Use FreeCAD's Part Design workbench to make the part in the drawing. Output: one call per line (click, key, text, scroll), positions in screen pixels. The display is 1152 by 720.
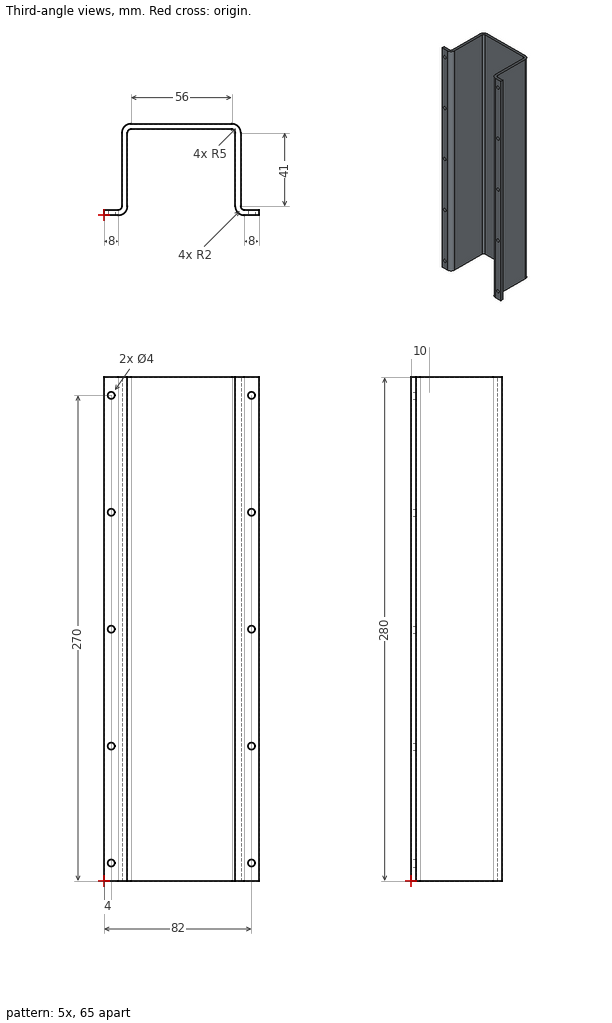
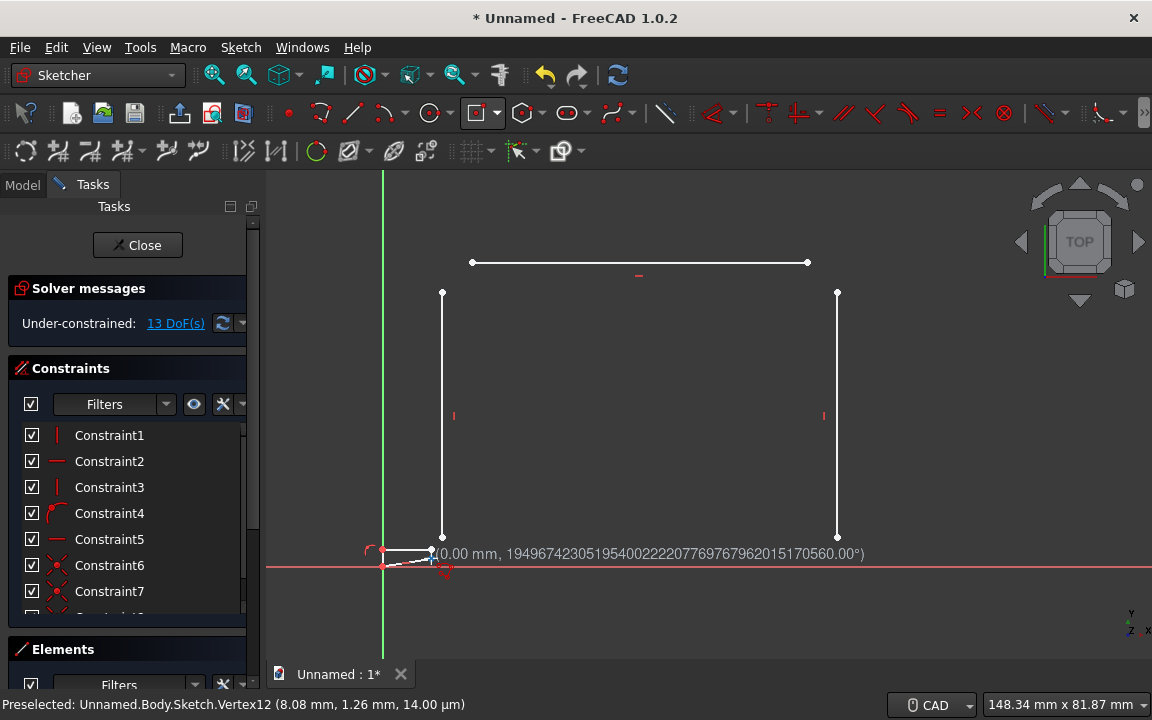
key(g)
key(l)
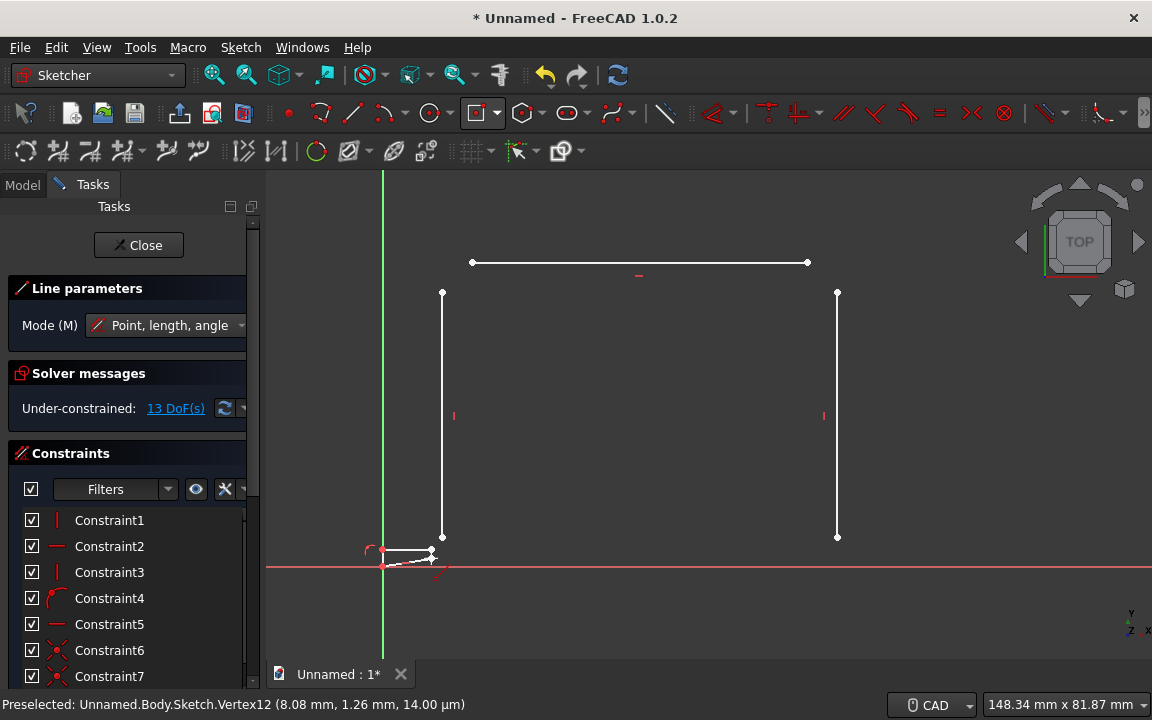
click(460, 537)
click(460, 292)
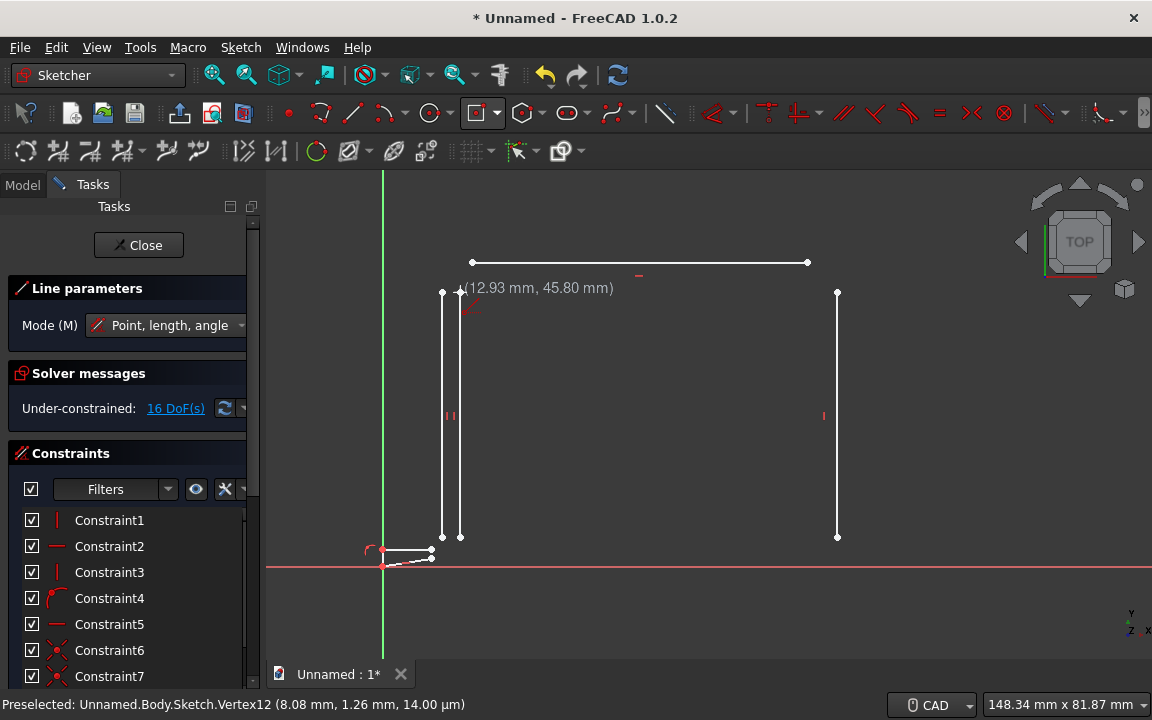
click(472, 280)
click(807, 280)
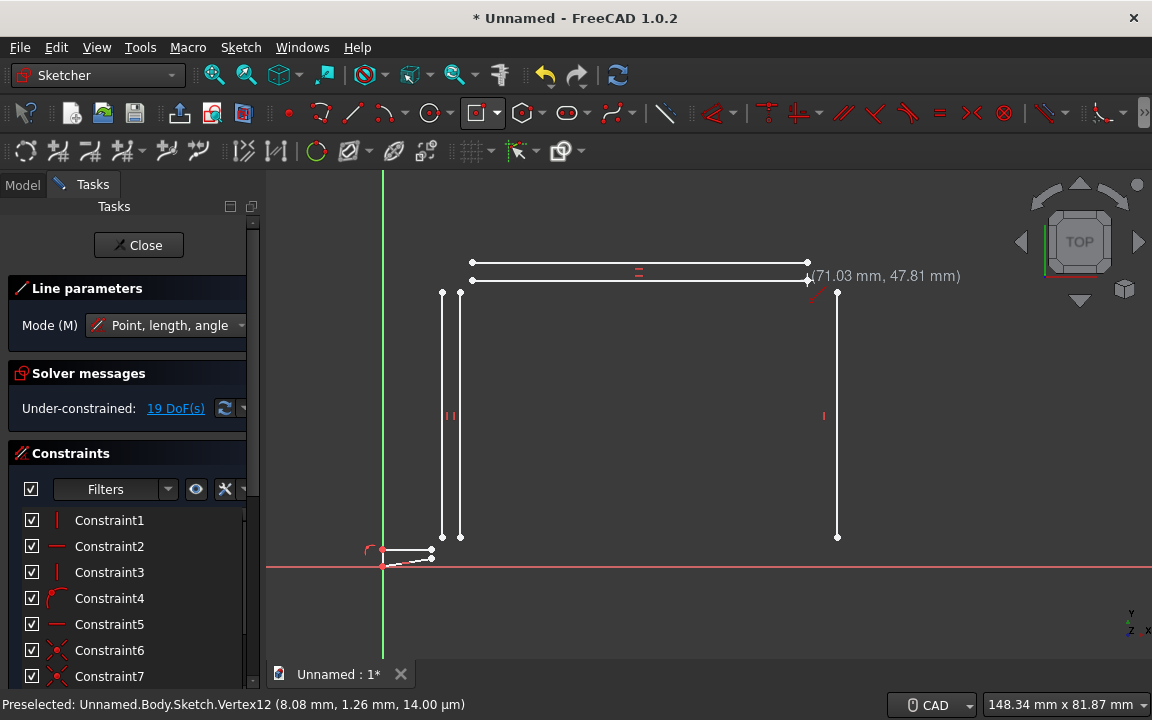
click(819, 292)
click(819, 537)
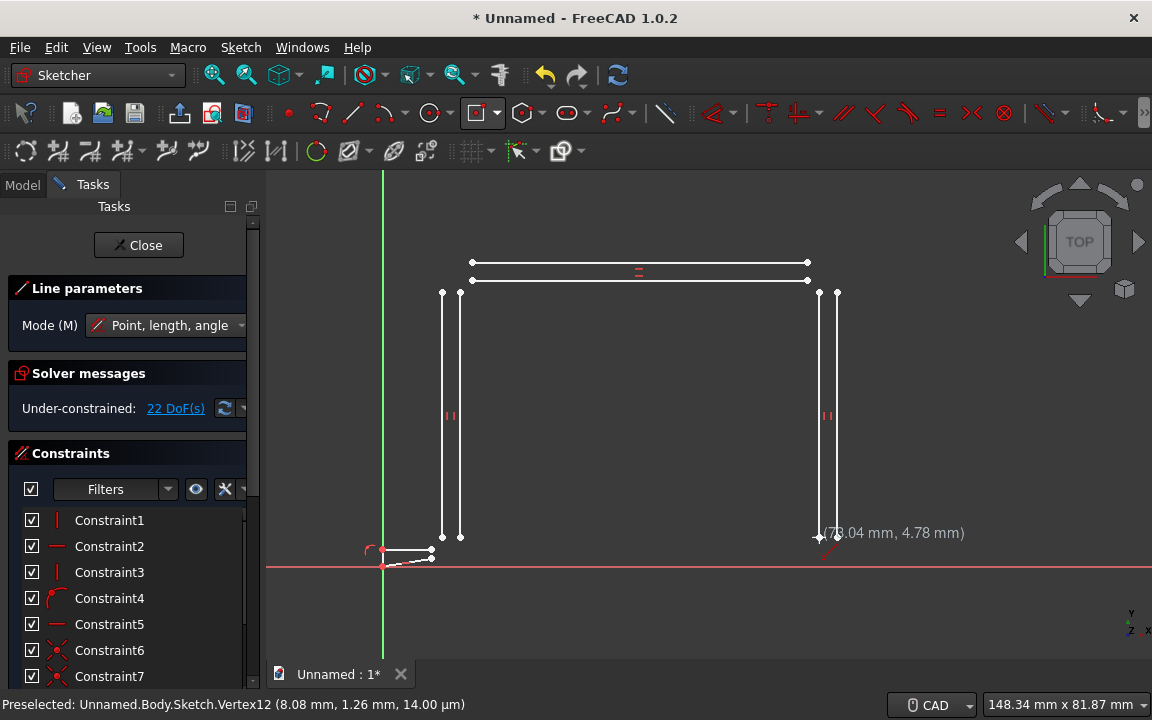
key(g)
key(m)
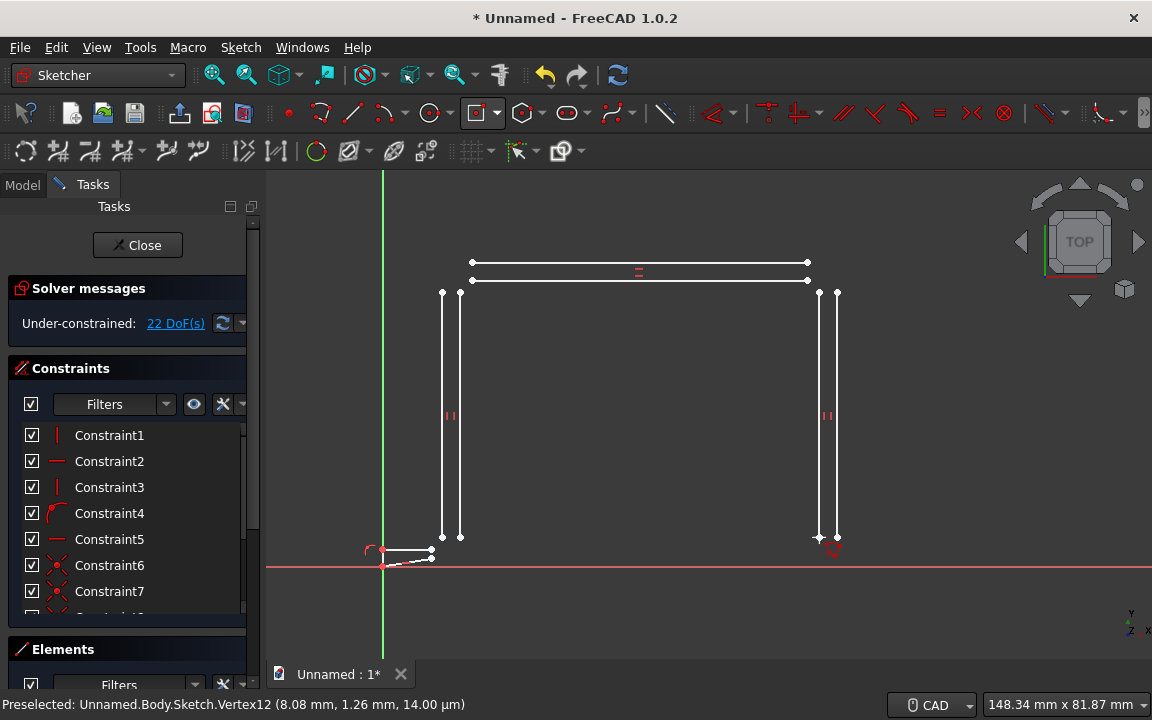
click(849, 567)
click(896, 558)
click(896, 549)
click(849, 549)
right_click(849, 549)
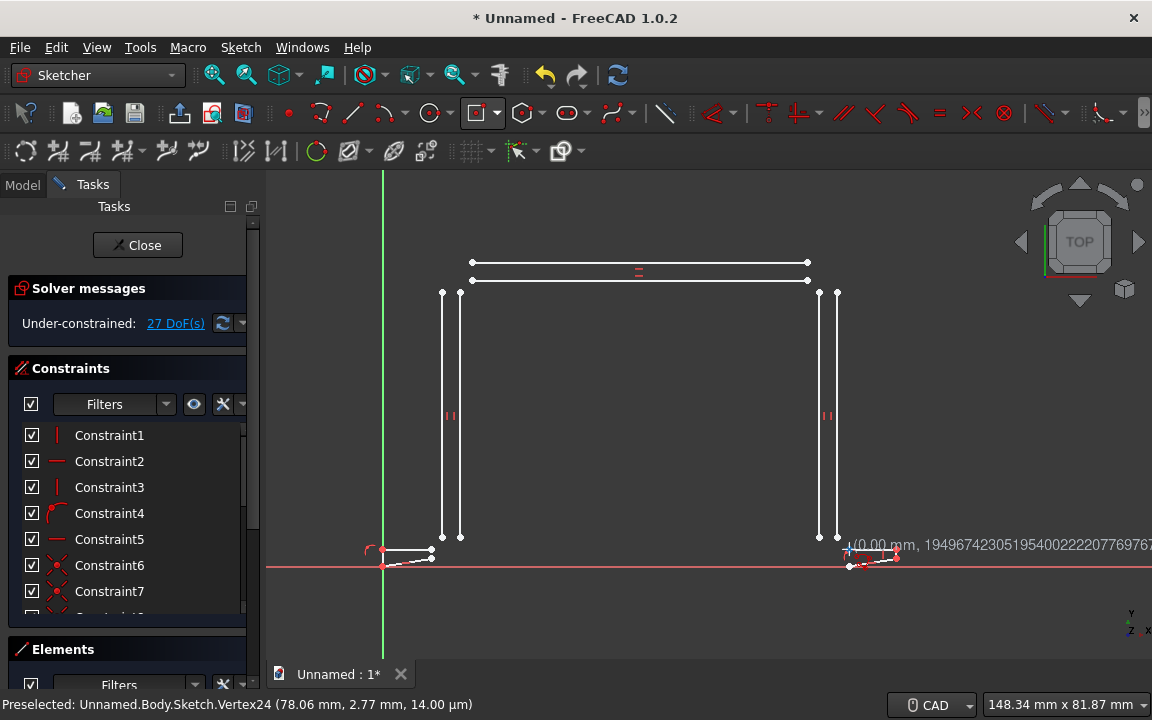
key(g)
key(3)
key(a)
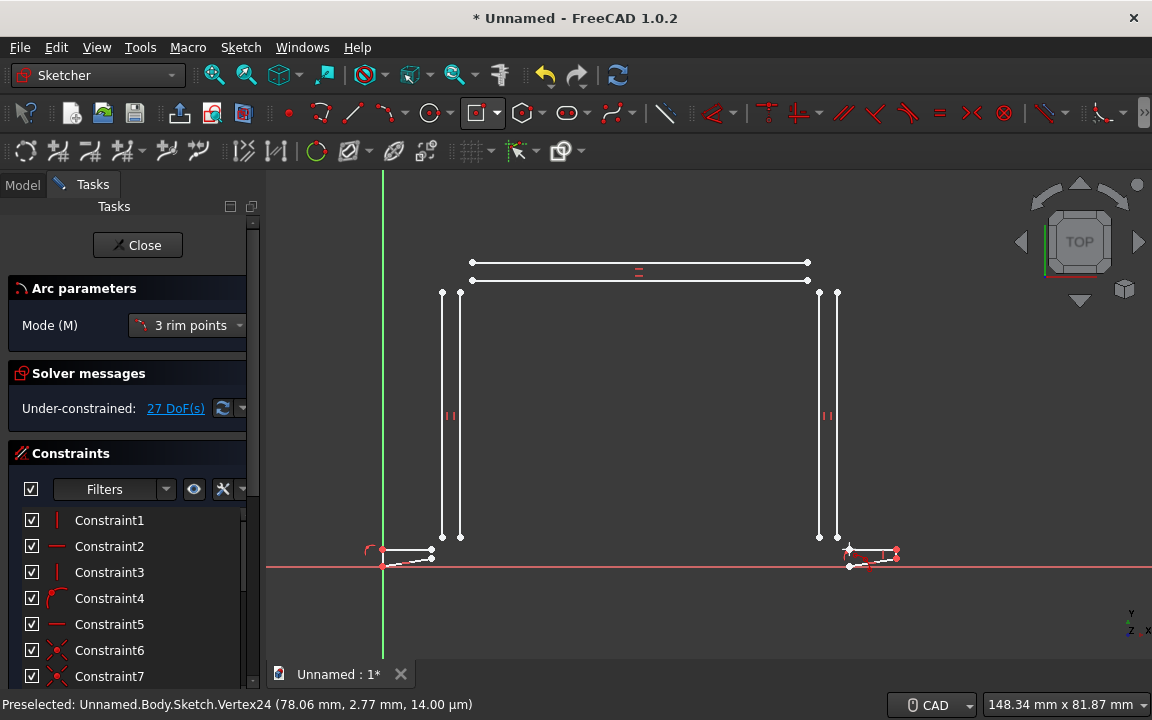
click(837, 293)
click(807, 263)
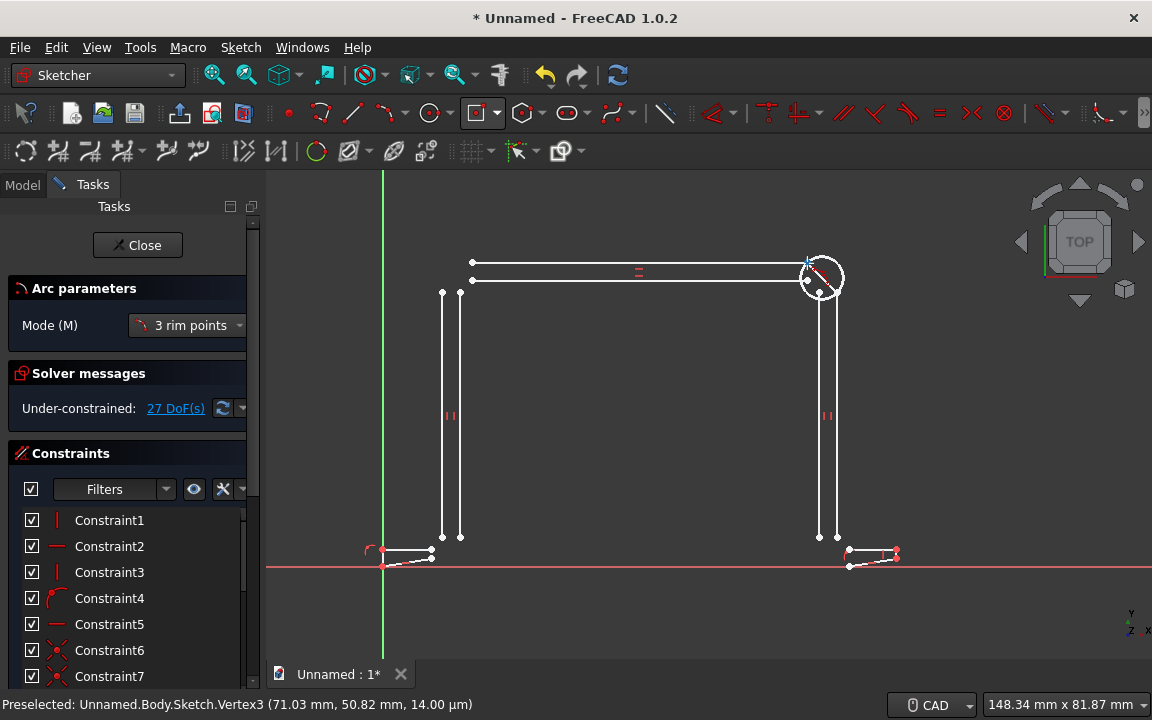
scroll(828, 271, up, 3)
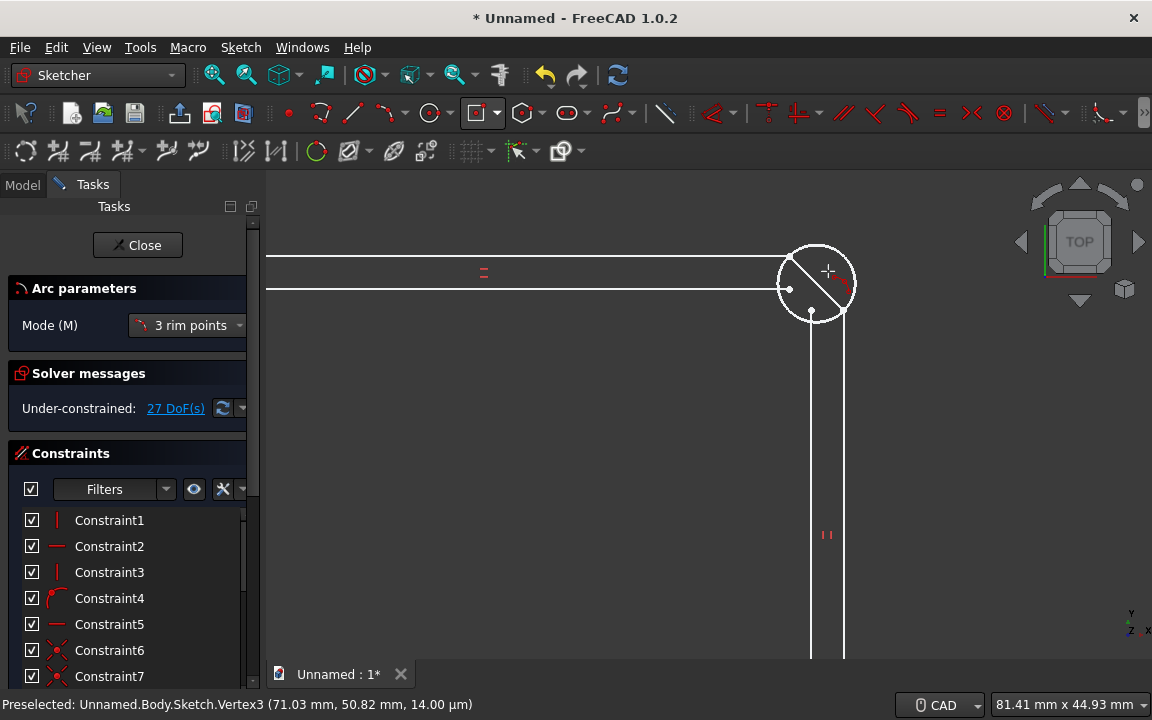
click(827, 270)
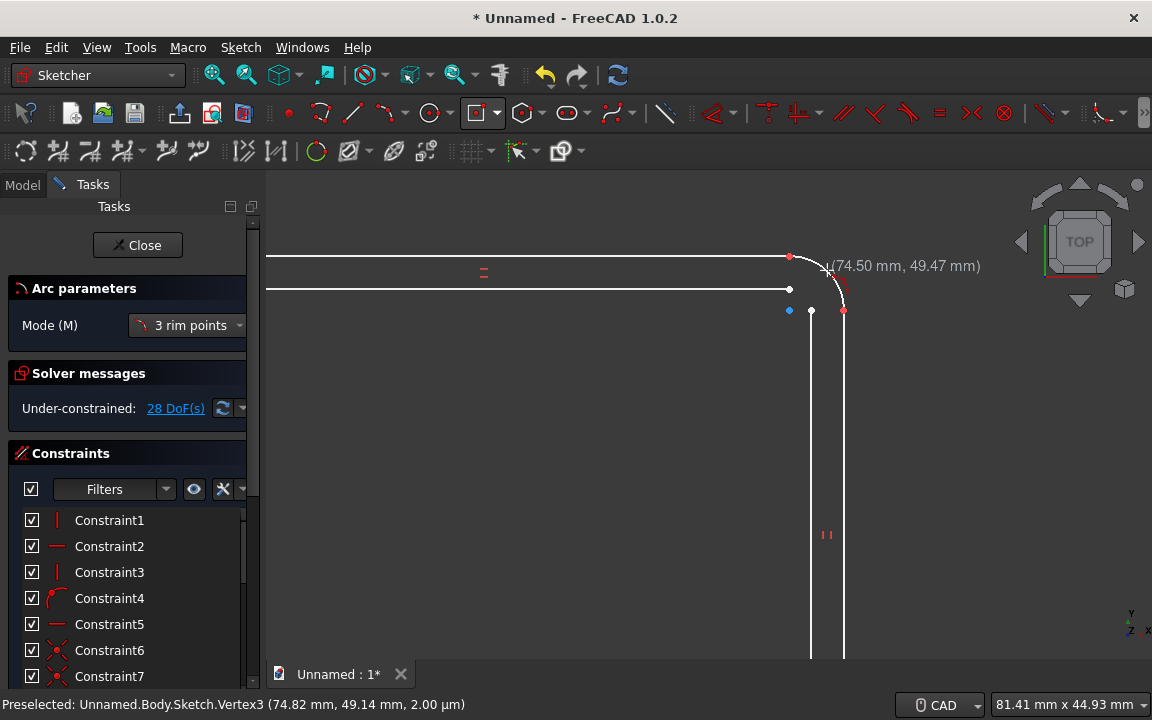
scroll(831, 272, down, 3)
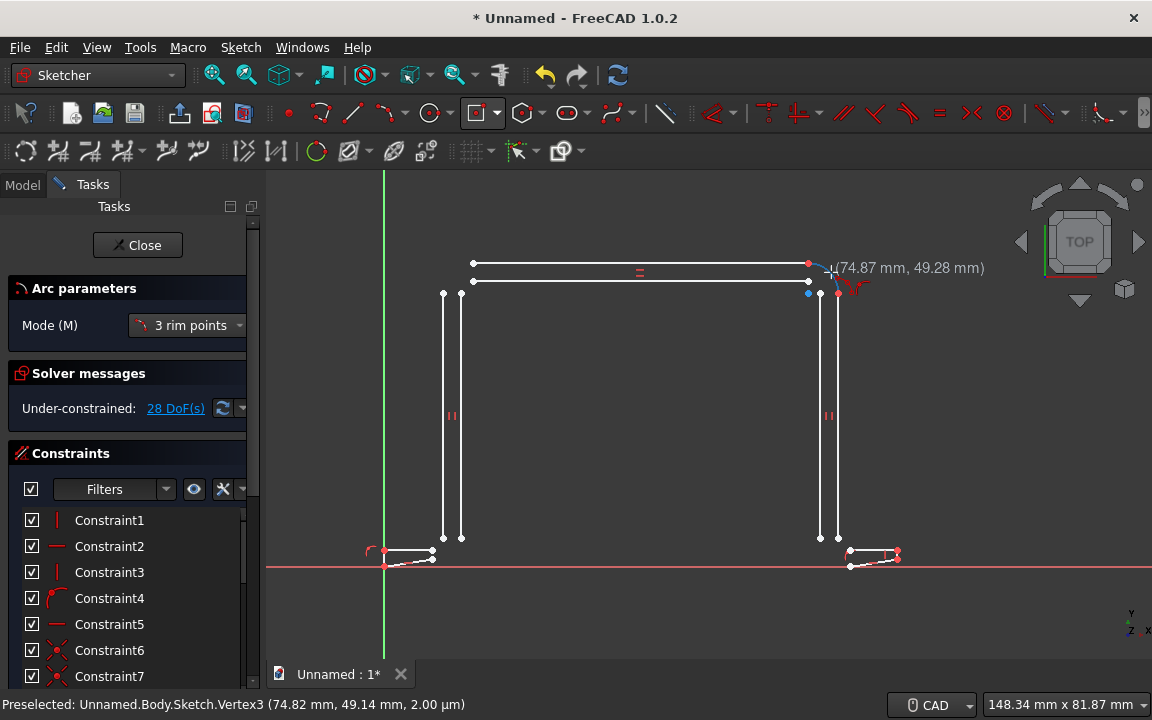
click(473, 263)
click(443, 293)